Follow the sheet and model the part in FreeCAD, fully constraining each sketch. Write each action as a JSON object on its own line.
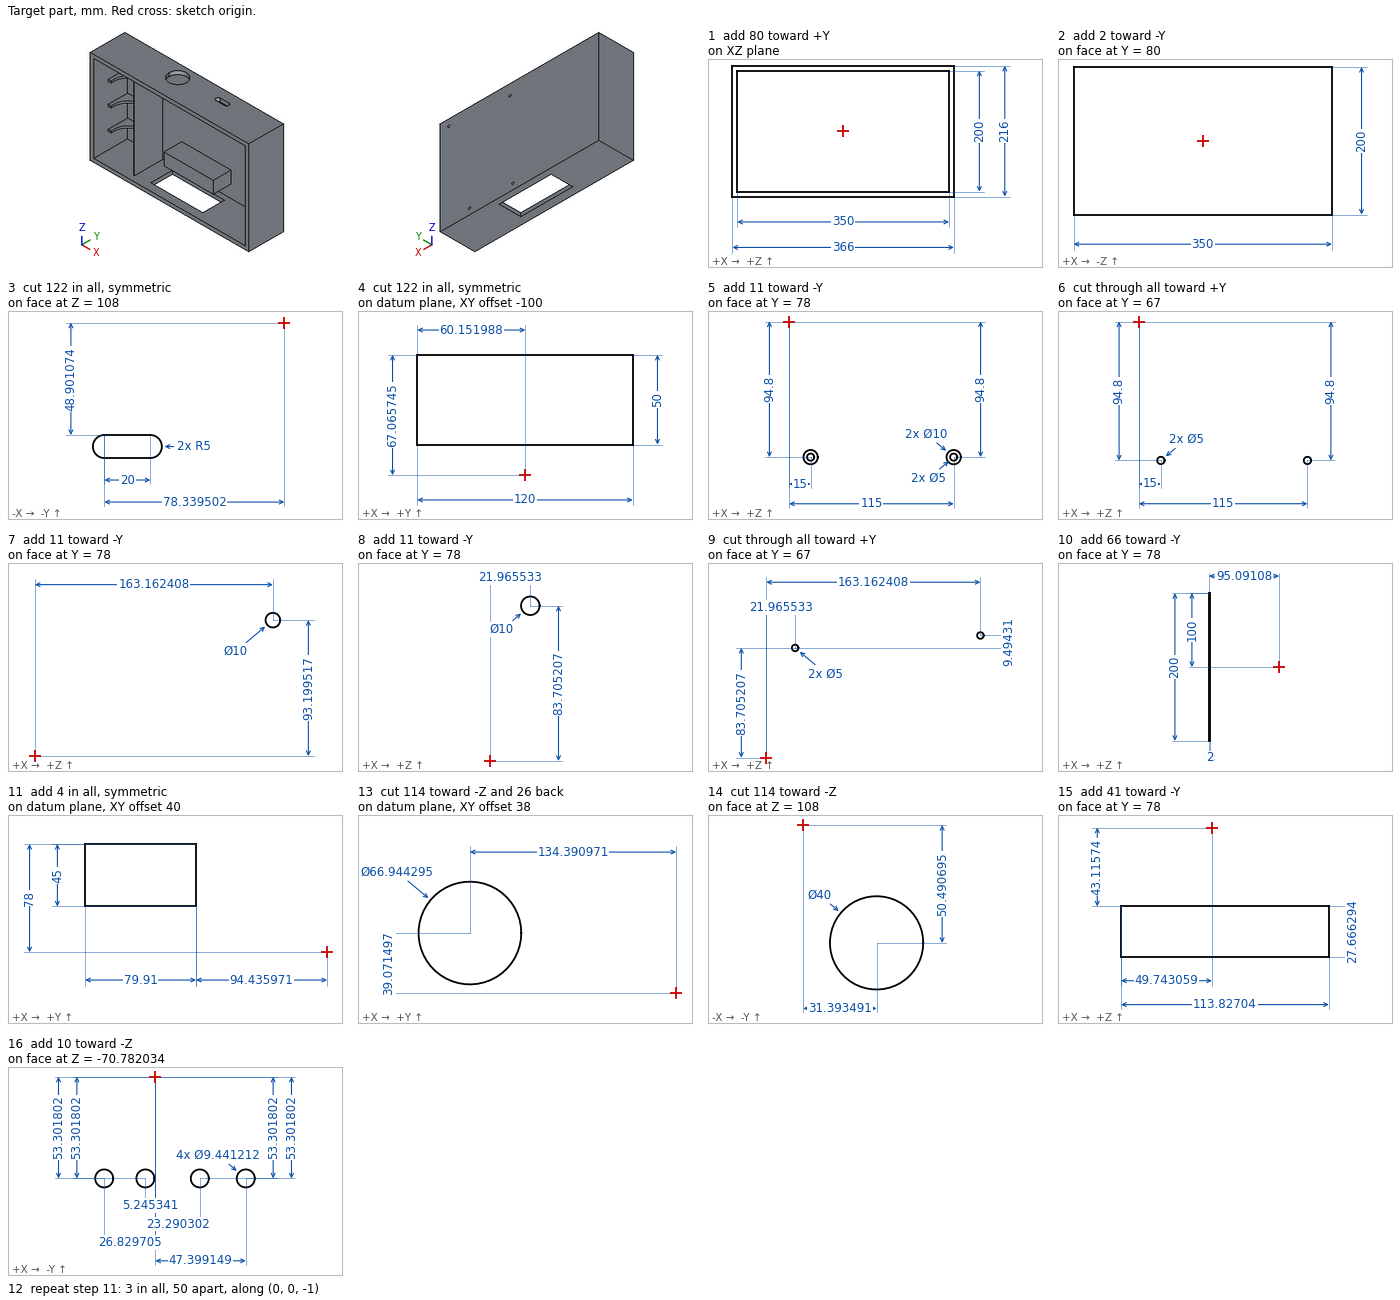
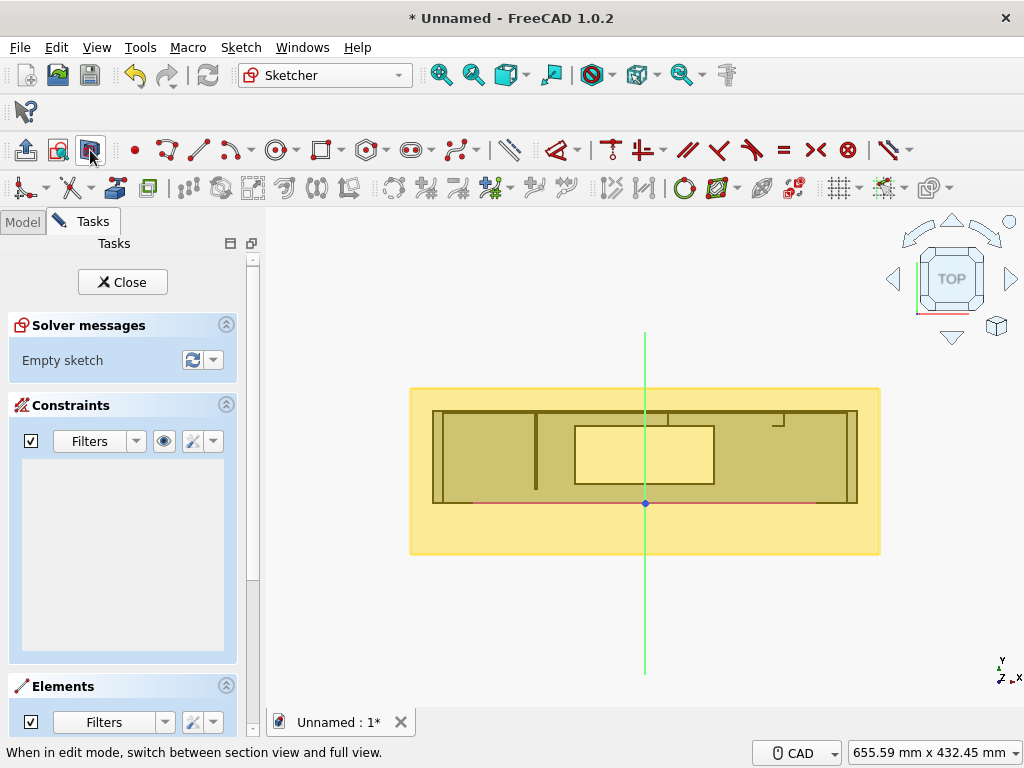
{"action": "scroll", "coordinate": [505, 460], "scroll_direction": "up", "scroll_amount": 3}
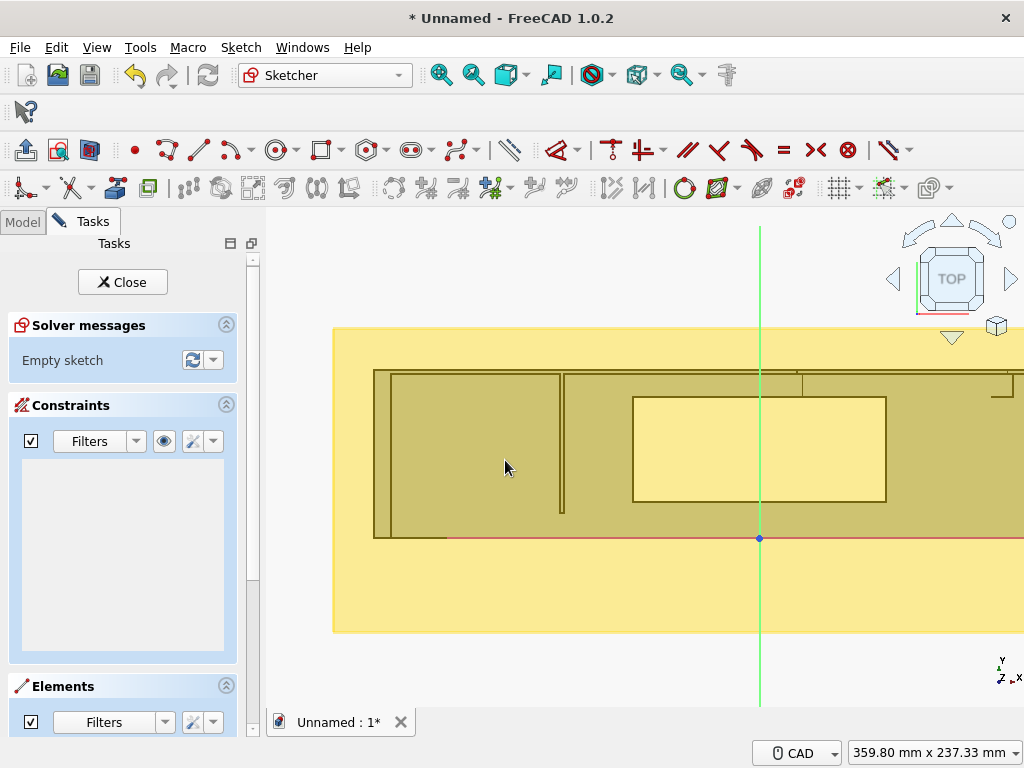
{"action": "key", "text": "g r"}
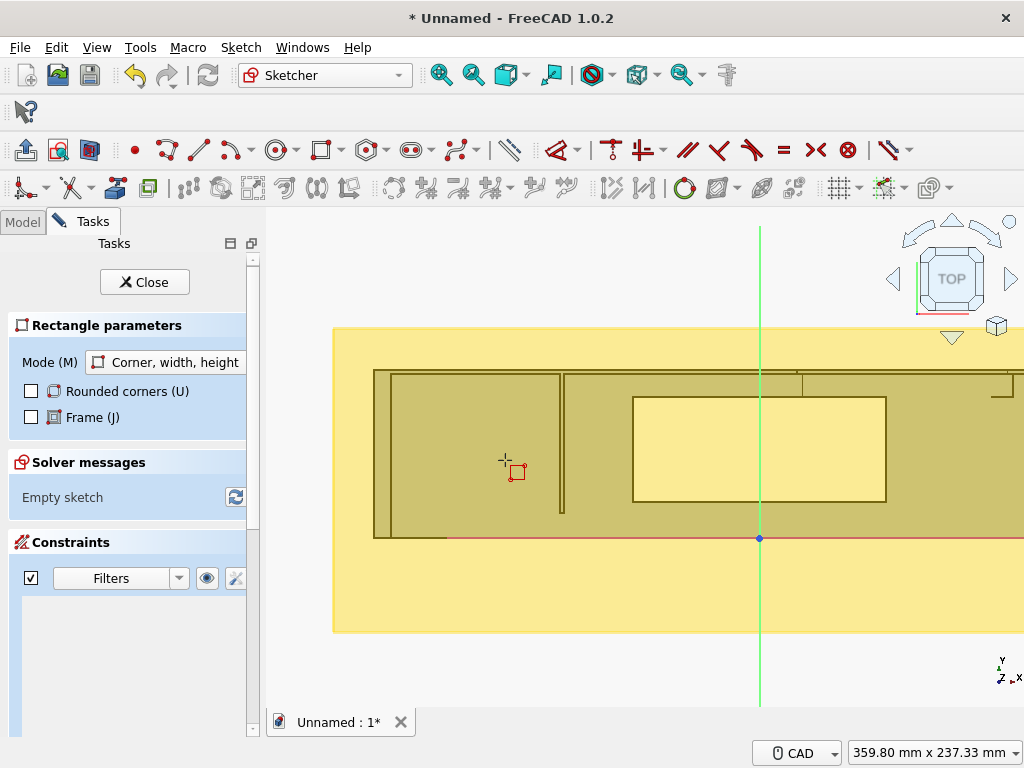
{"action": "left_click", "coordinate": [393, 374]}
{"action": "mouse_move", "coordinate": [561, 469]}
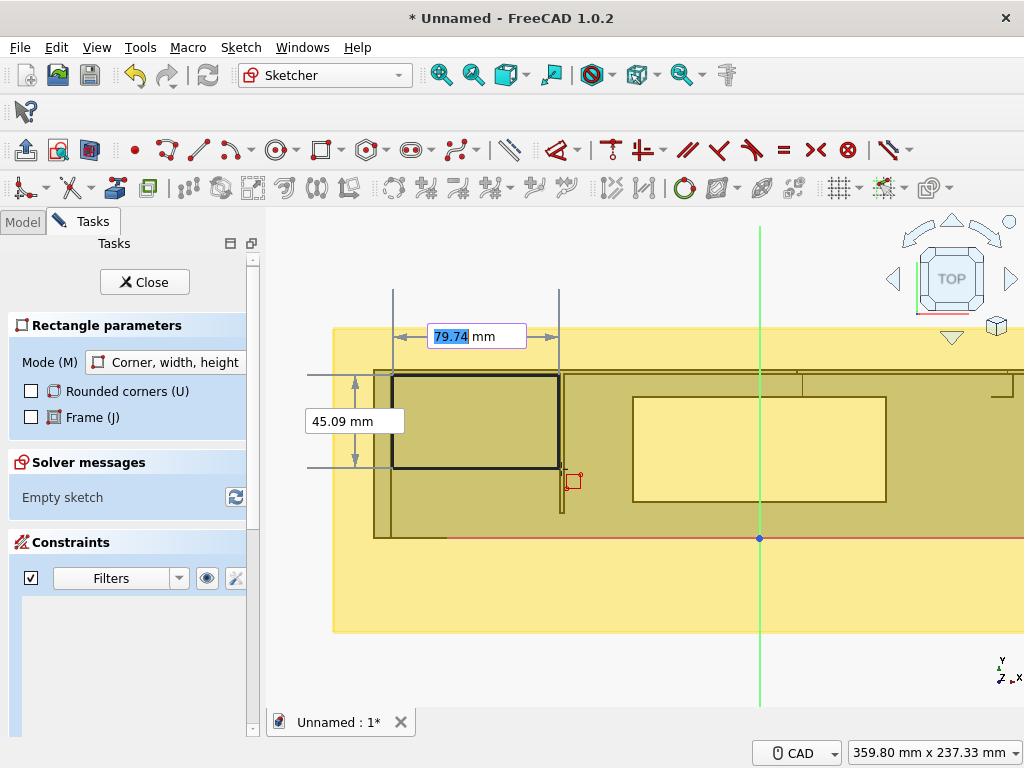
{"action": "type", "text": "79.91"}
{"action": "key", "text": "Tab"}
{"action": "type", "text": "45"}
{"action": "key", "text": "Return"}
{"action": "key", "text": "Escape"}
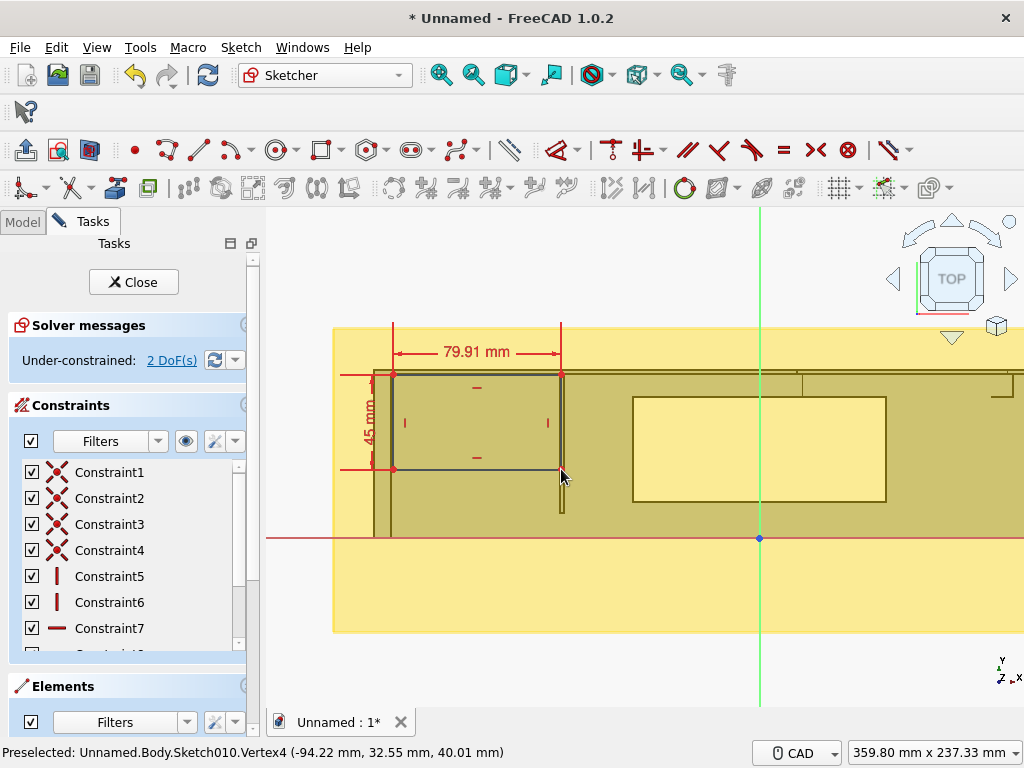
{"action": "key", "text": "d"}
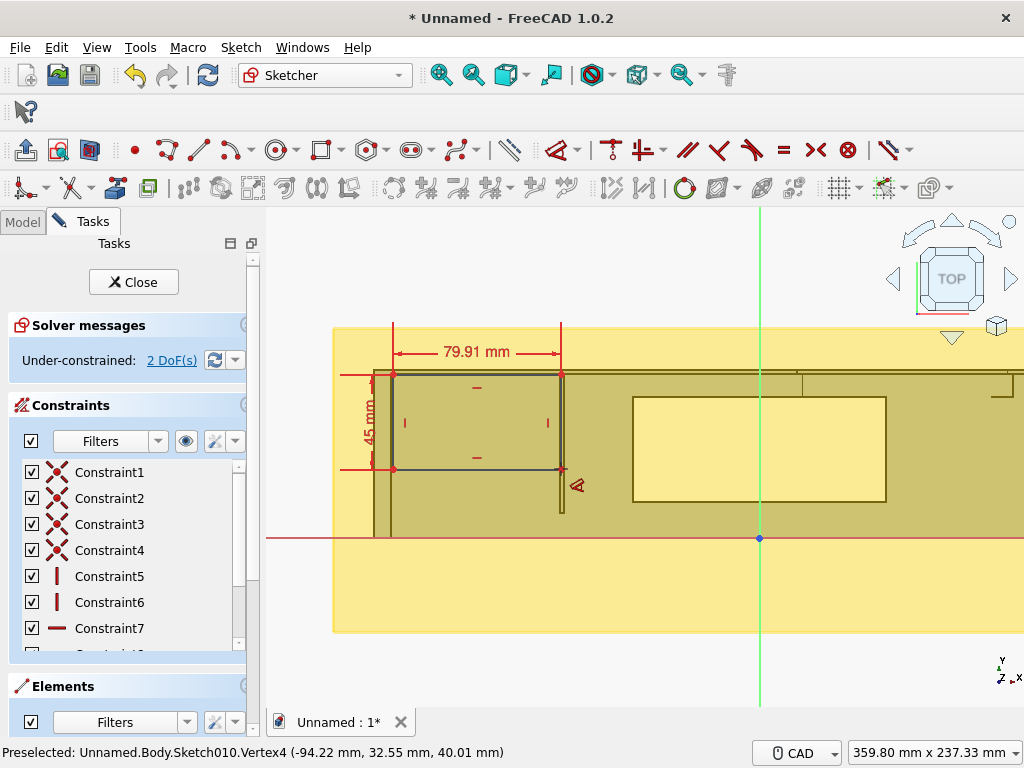
{"action": "left_click", "coordinate": [393, 375]}
{"action": "left_click", "coordinate": [794, 457]}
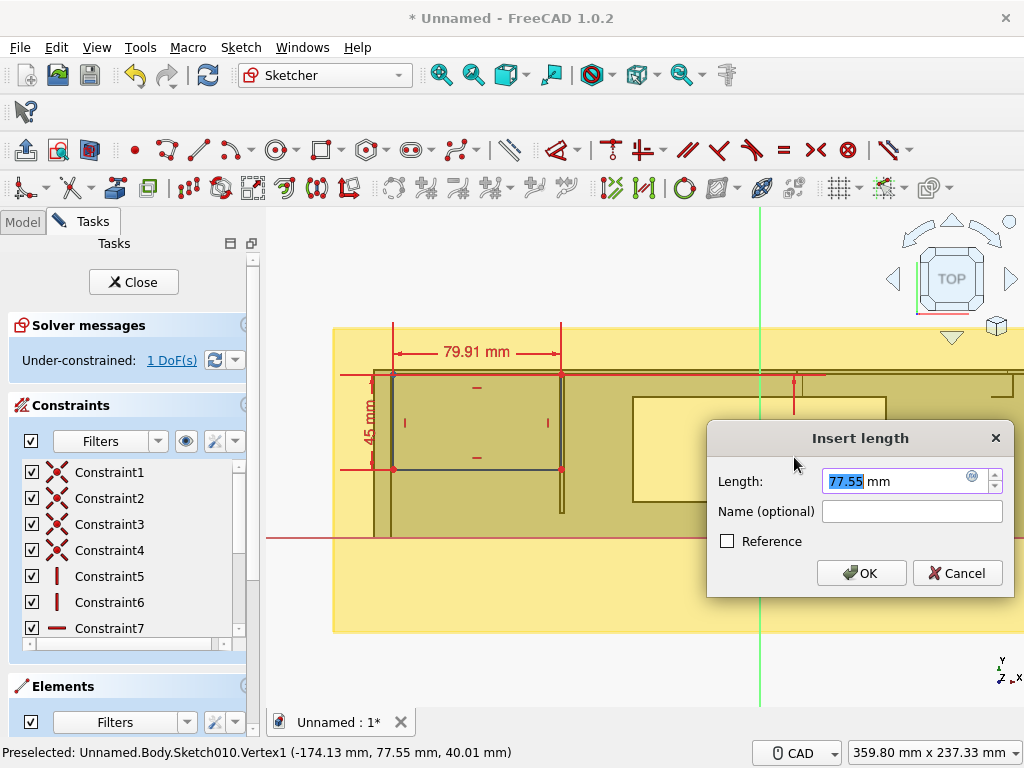
{"action": "type", "text": "78"}
{"action": "key", "text": "Return"}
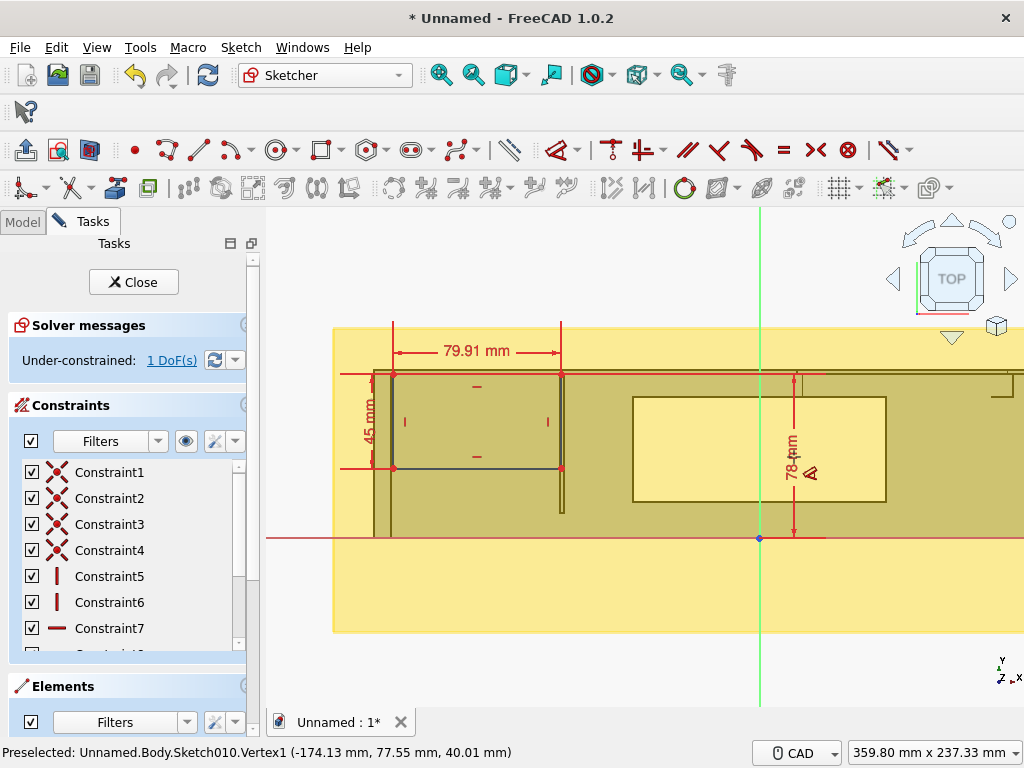
{"action": "left_click", "coordinate": [561, 469]}
{"action": "left_click", "coordinate": [661, 572]}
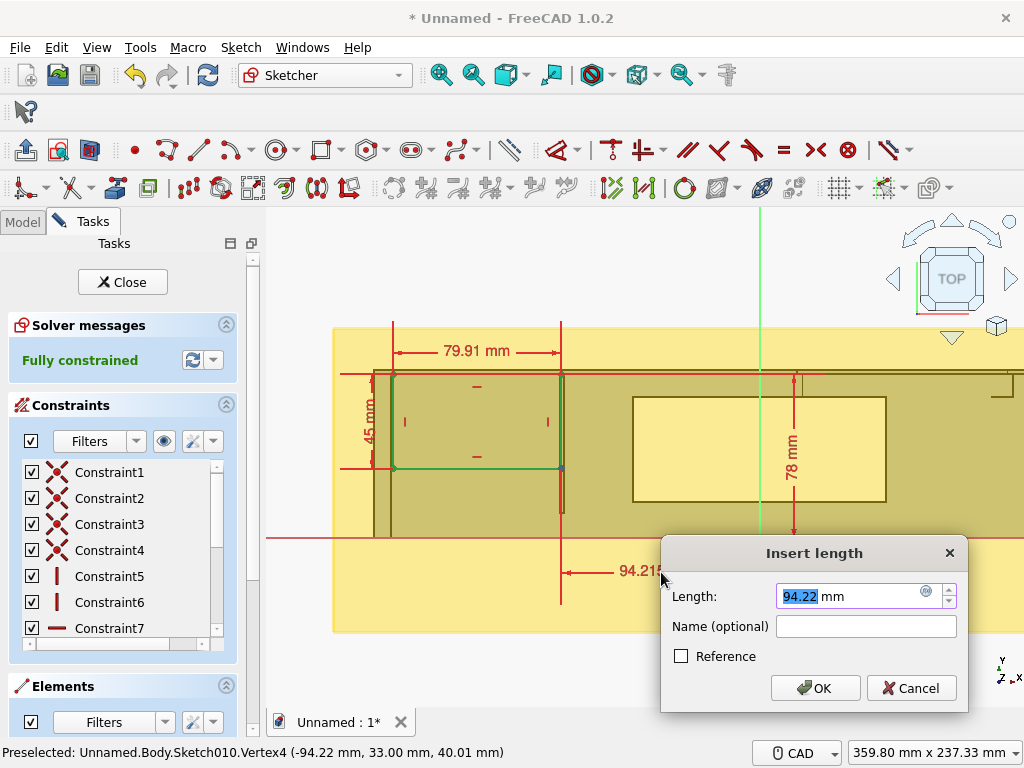
{"action": "type", "text": "94.435971"}
{"action": "key", "text": "Return"}
{"action": "key", "text": "Escape"}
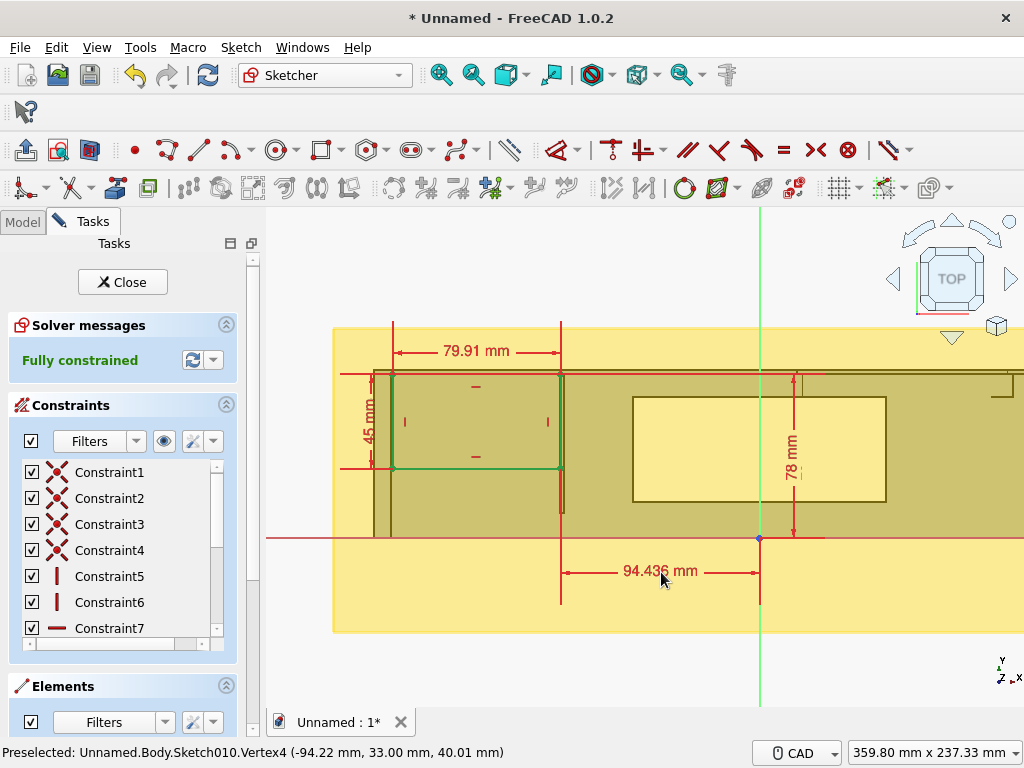
{"action": "left_click", "coordinate": [123, 282]}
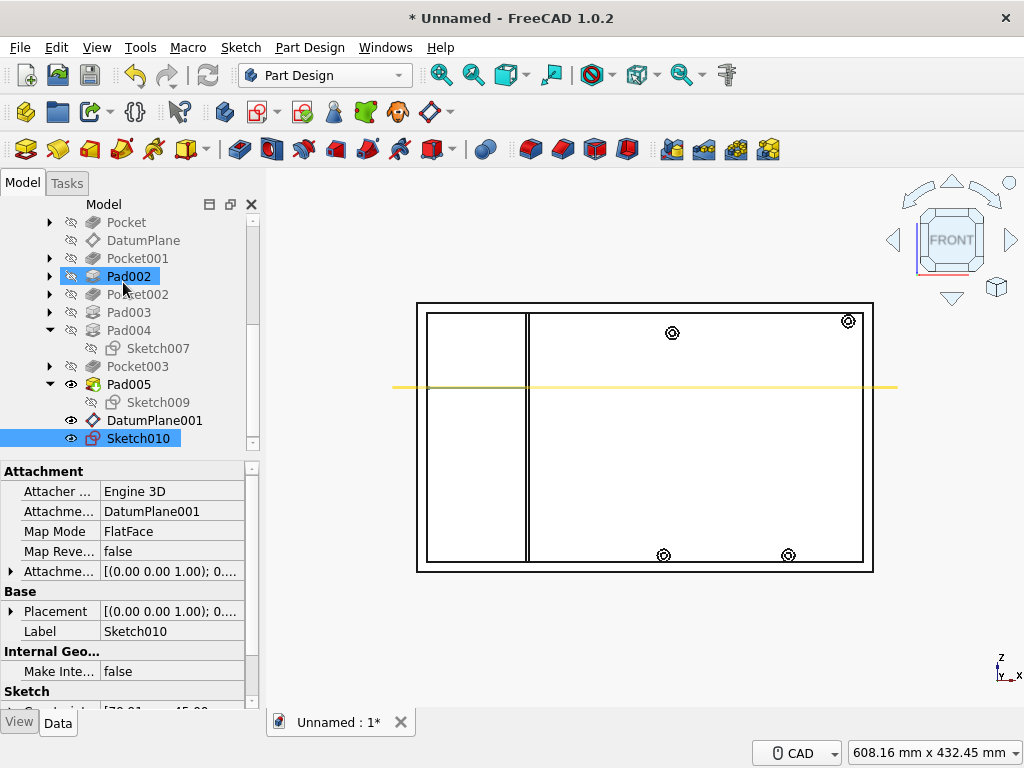
{"action": "left_click", "coordinate": [26, 150]}